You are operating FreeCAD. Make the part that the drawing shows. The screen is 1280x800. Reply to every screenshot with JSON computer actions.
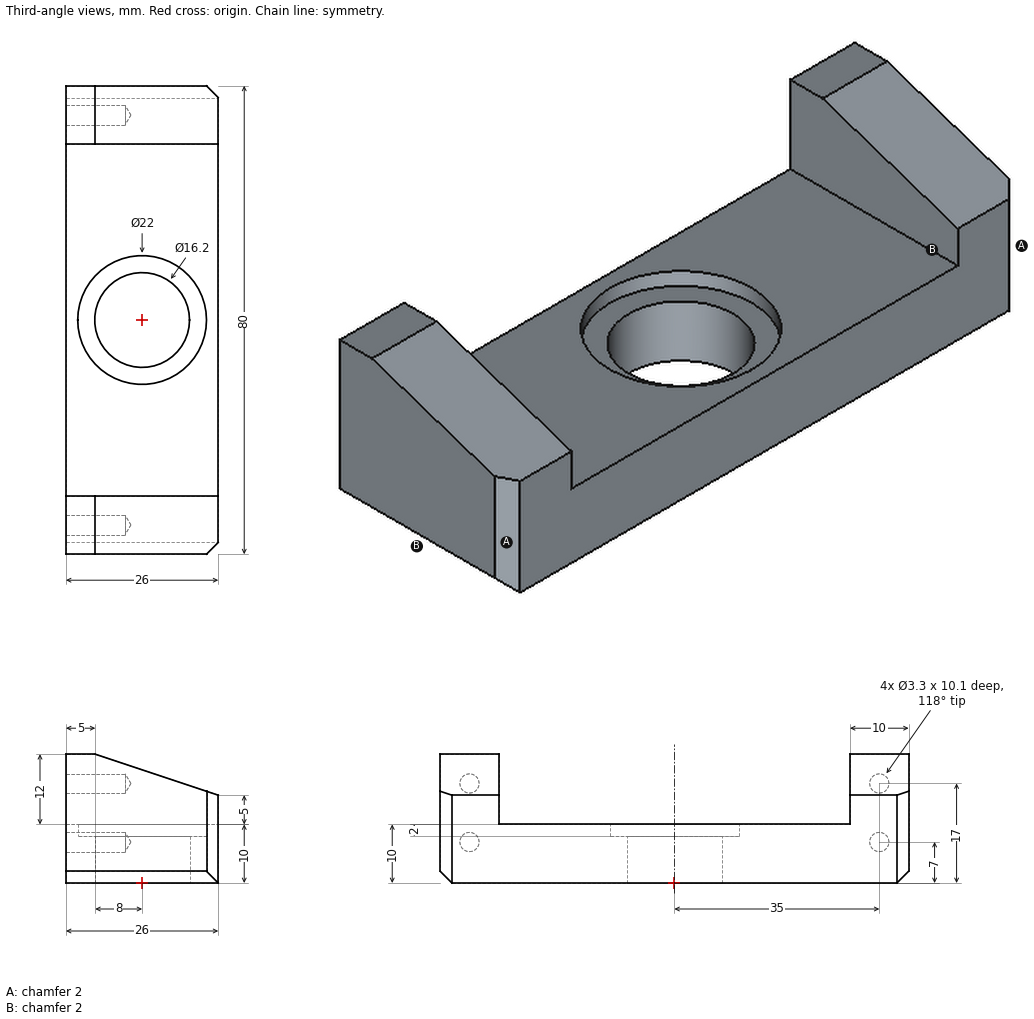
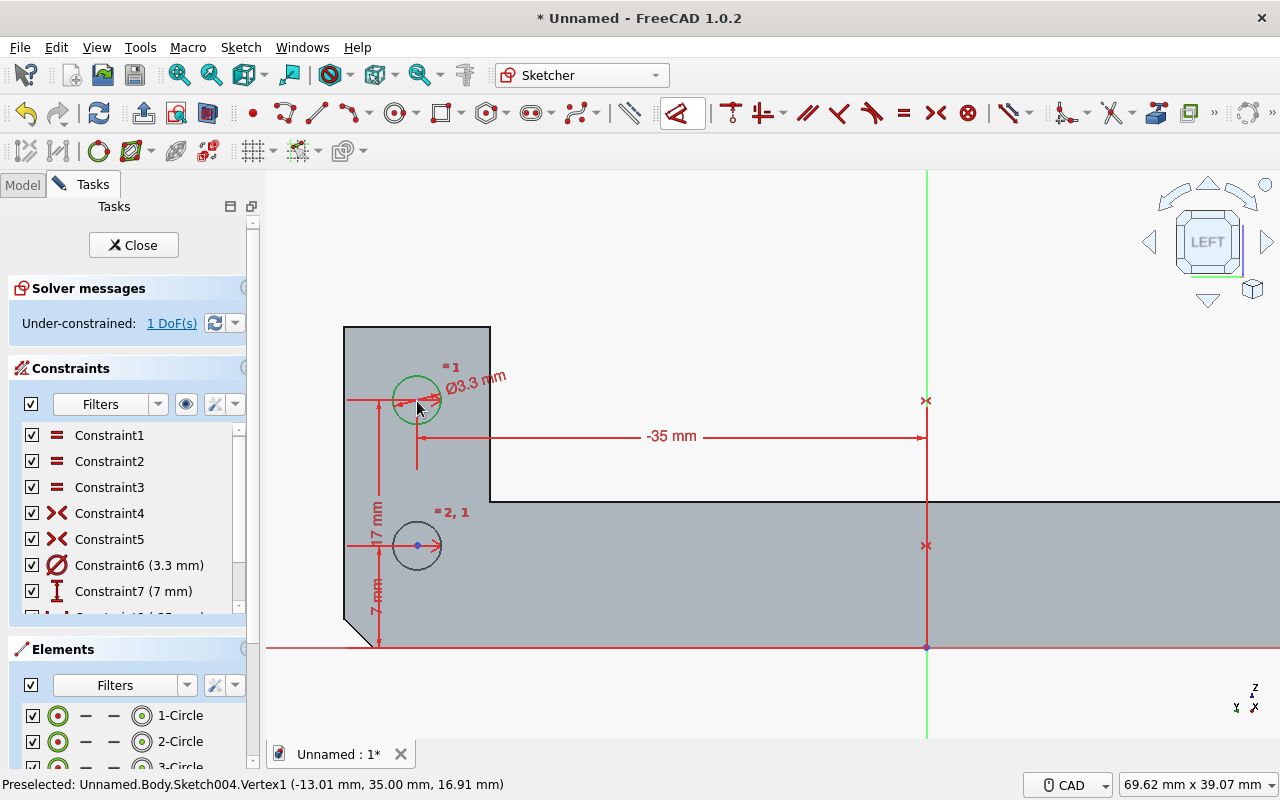
{"action": "left_click", "coordinate": [417, 546]}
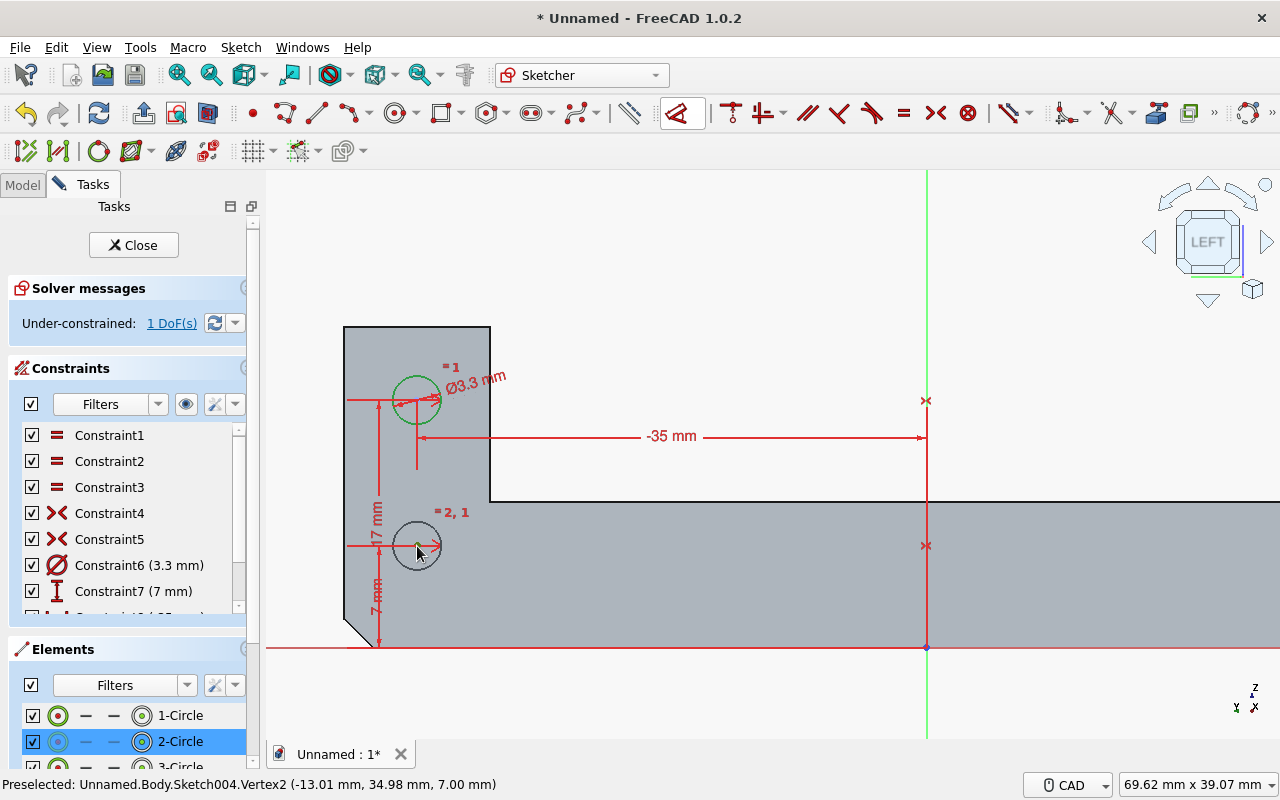
{"action": "key", "text": "l"}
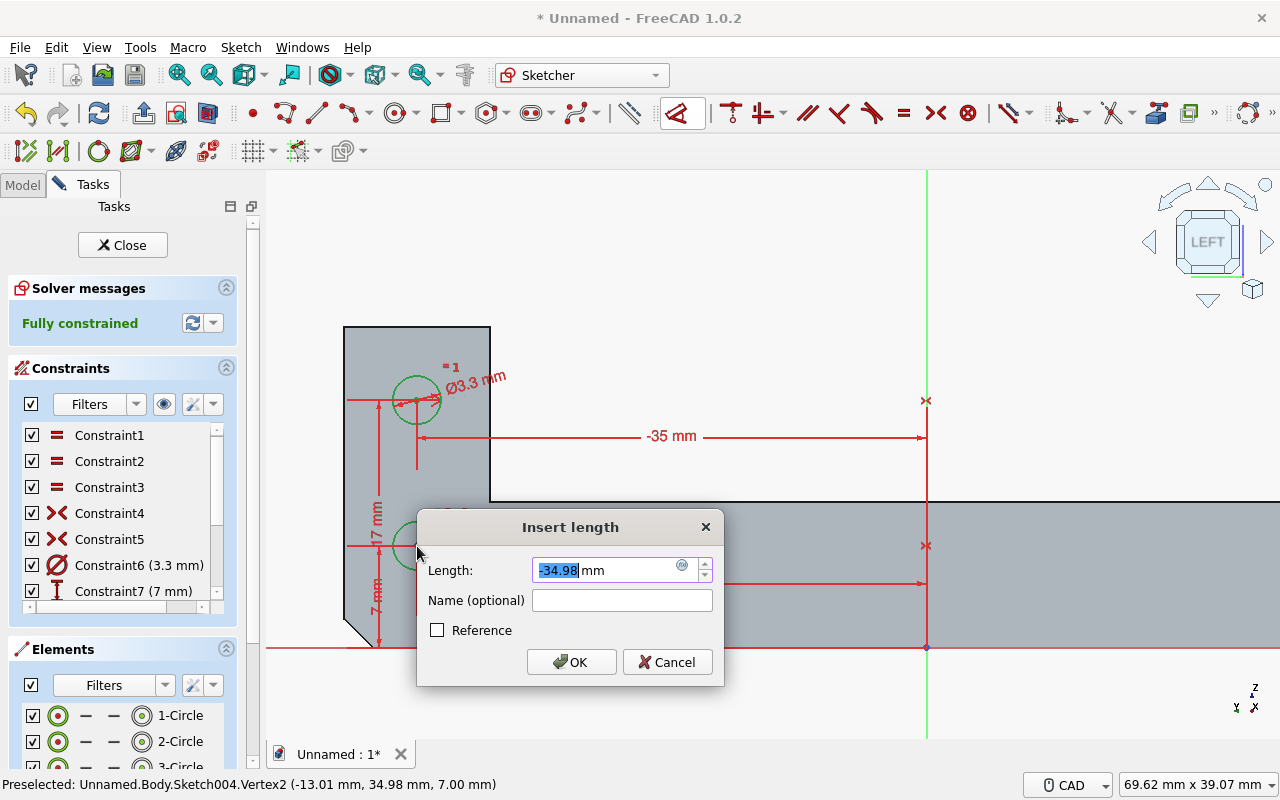
{"action": "type", "text": "-35"}
{"action": "key", "text": "Return"}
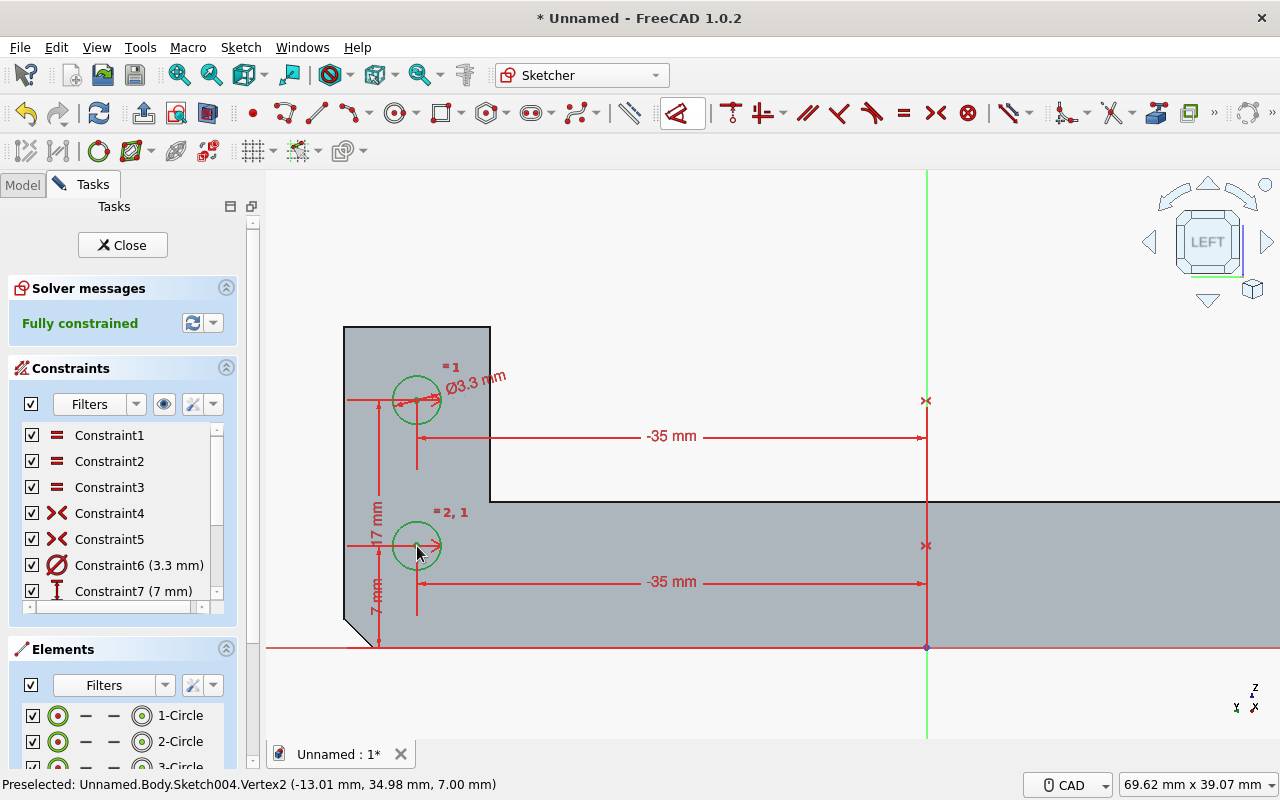
{"action": "left_click", "coordinate": [123, 245]}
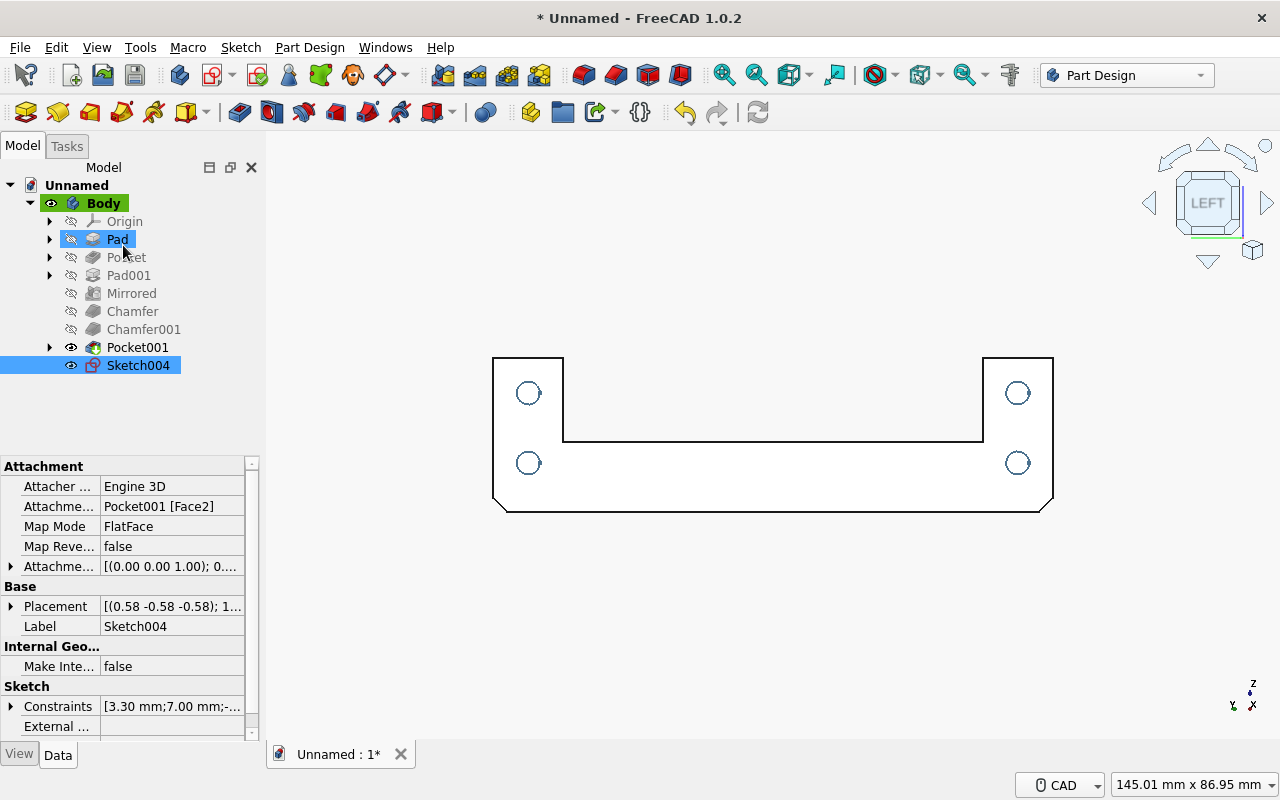
{"action": "left_click", "coordinate": [272, 112]}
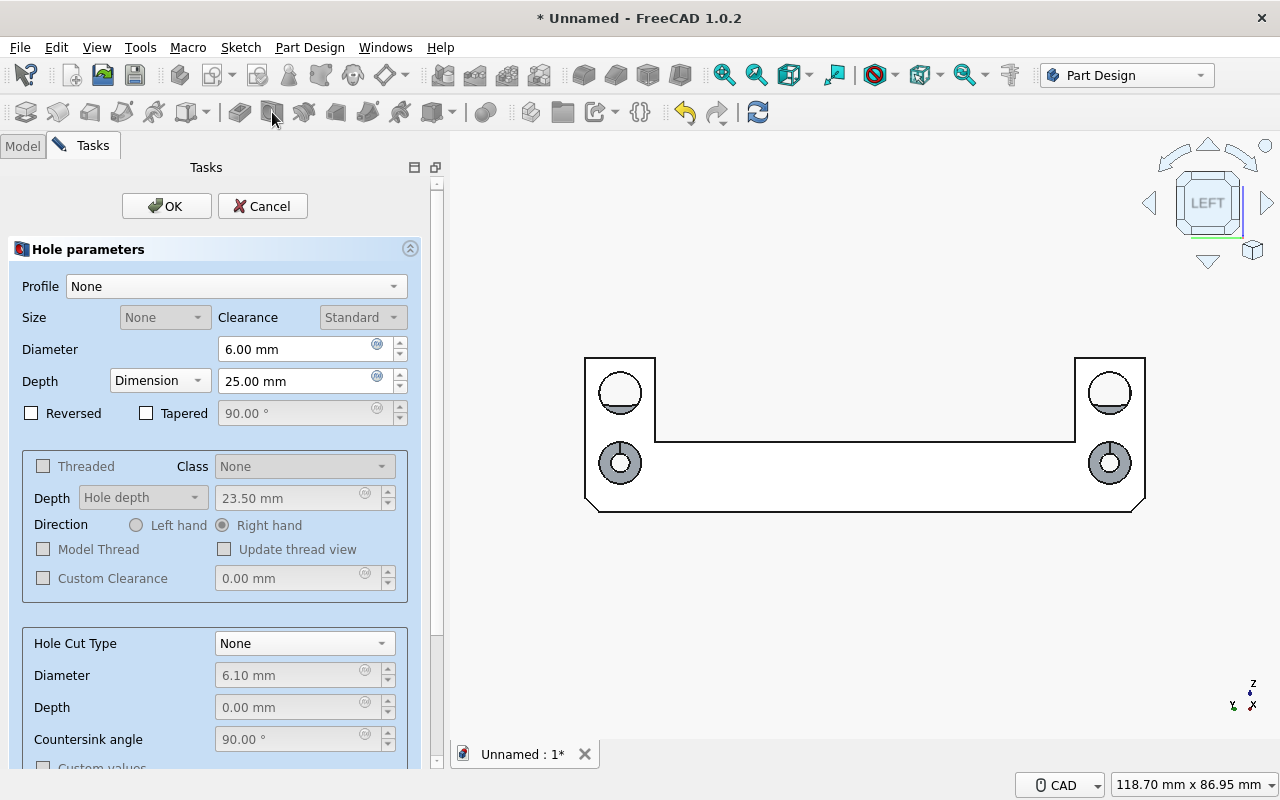
{"action": "triple_click", "coordinate": [305, 349]}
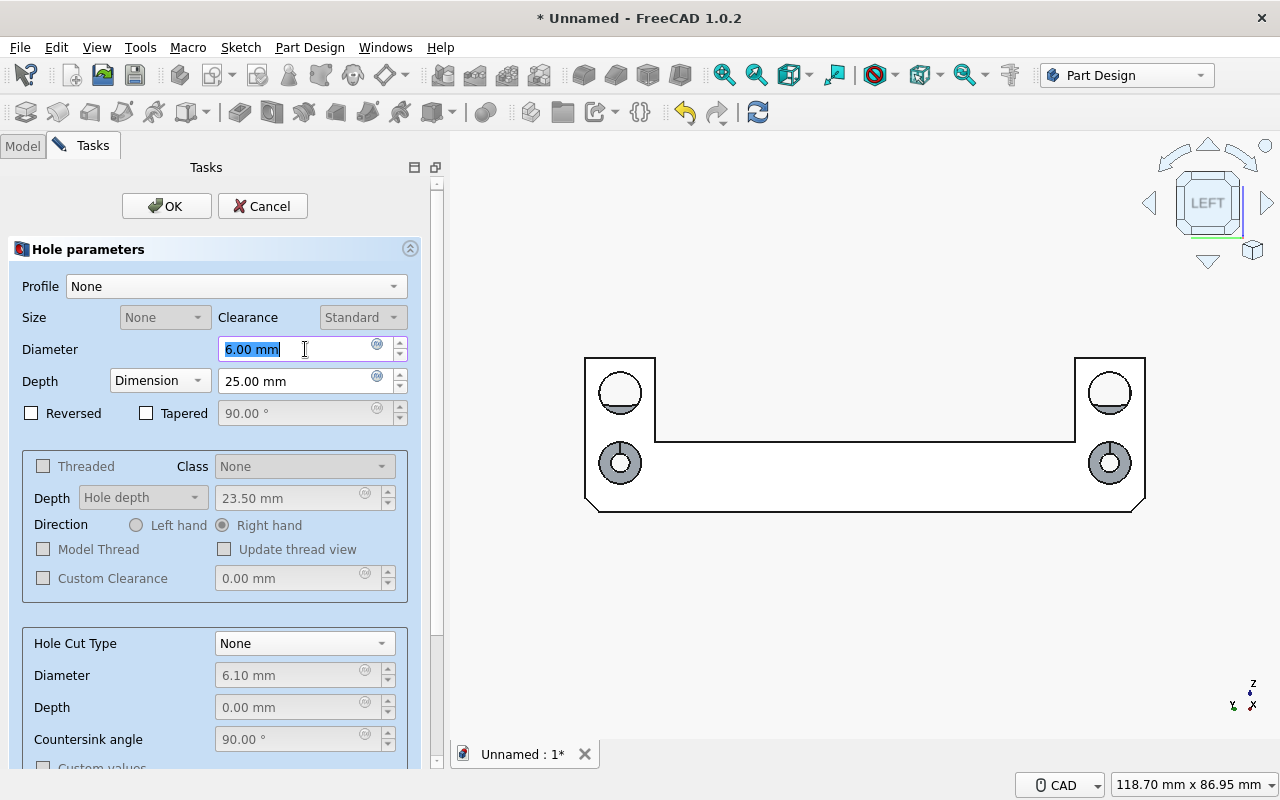
{"action": "type", "text": "3.3"}
{"action": "key", "text": "Tab"}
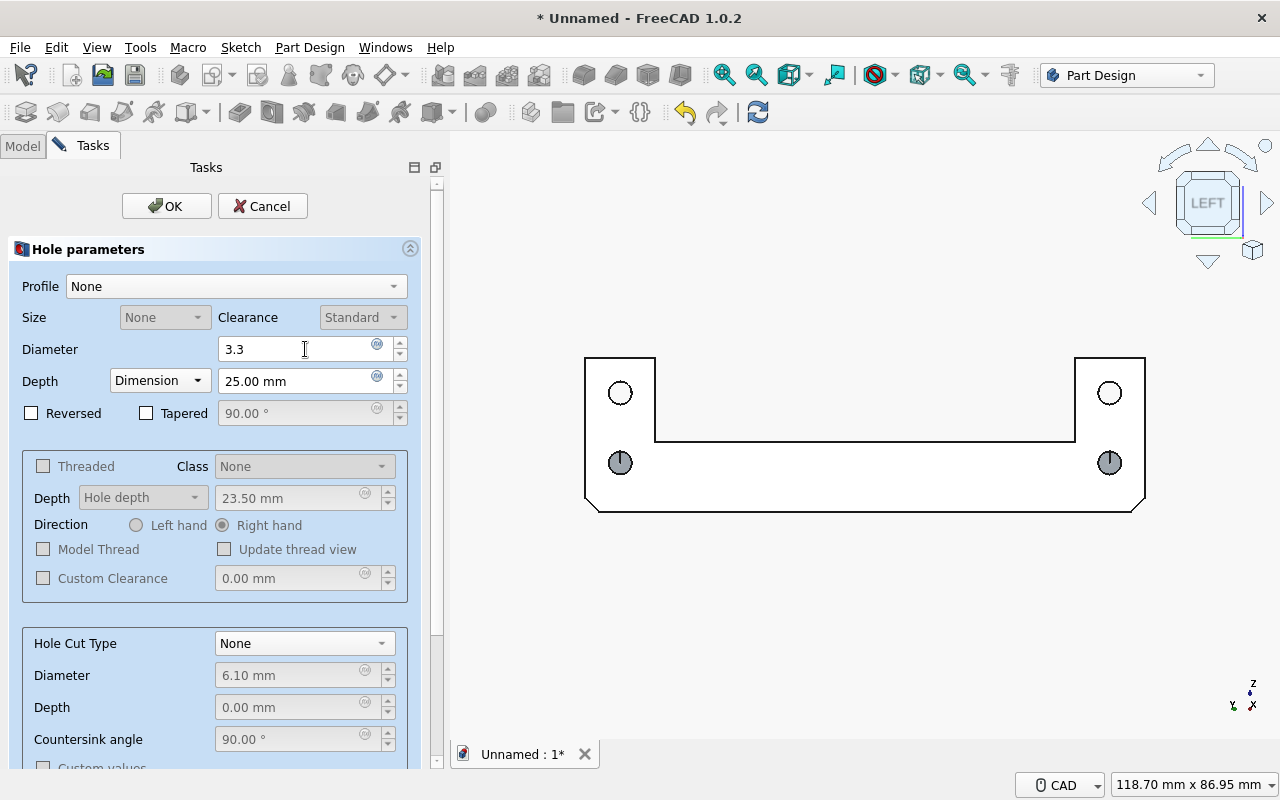
{"action": "triple_click", "coordinate": [305, 381]}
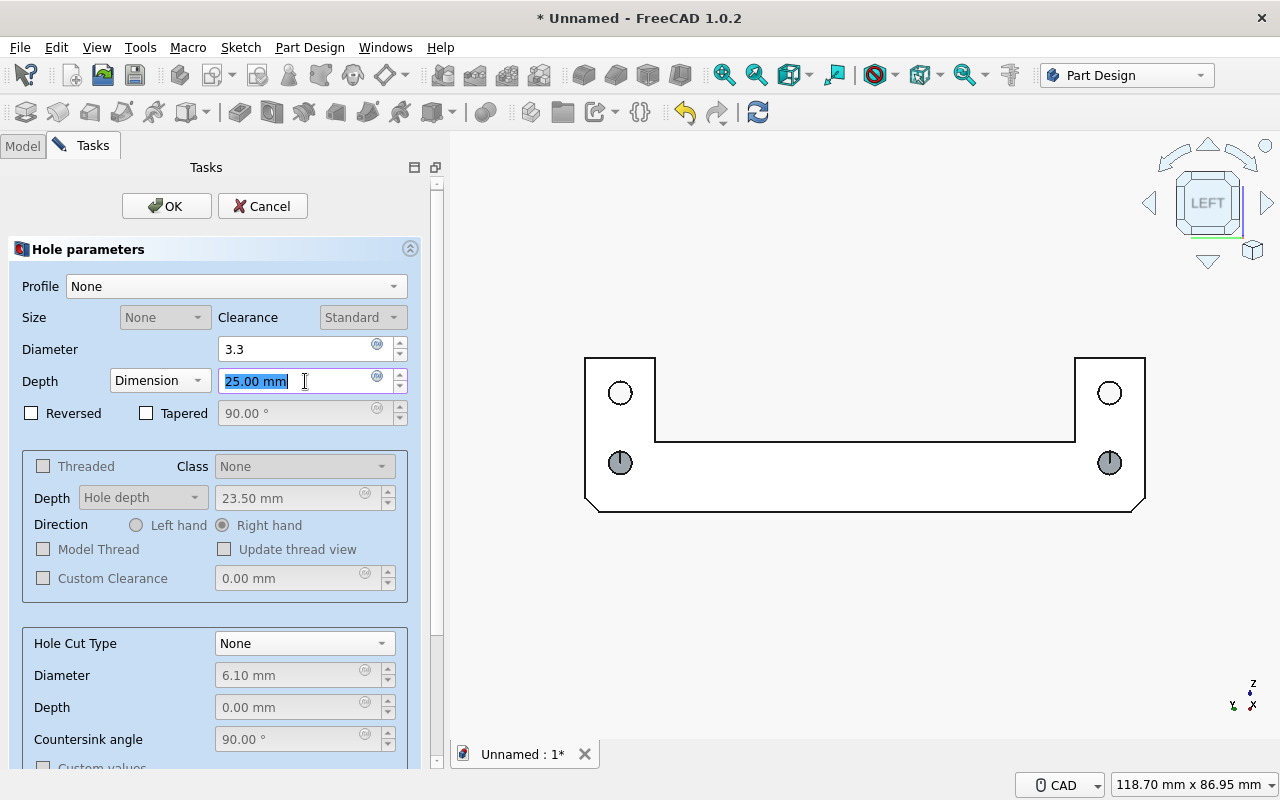
{"action": "type", "text": "10.1"}
{"action": "key", "text": "Tab"}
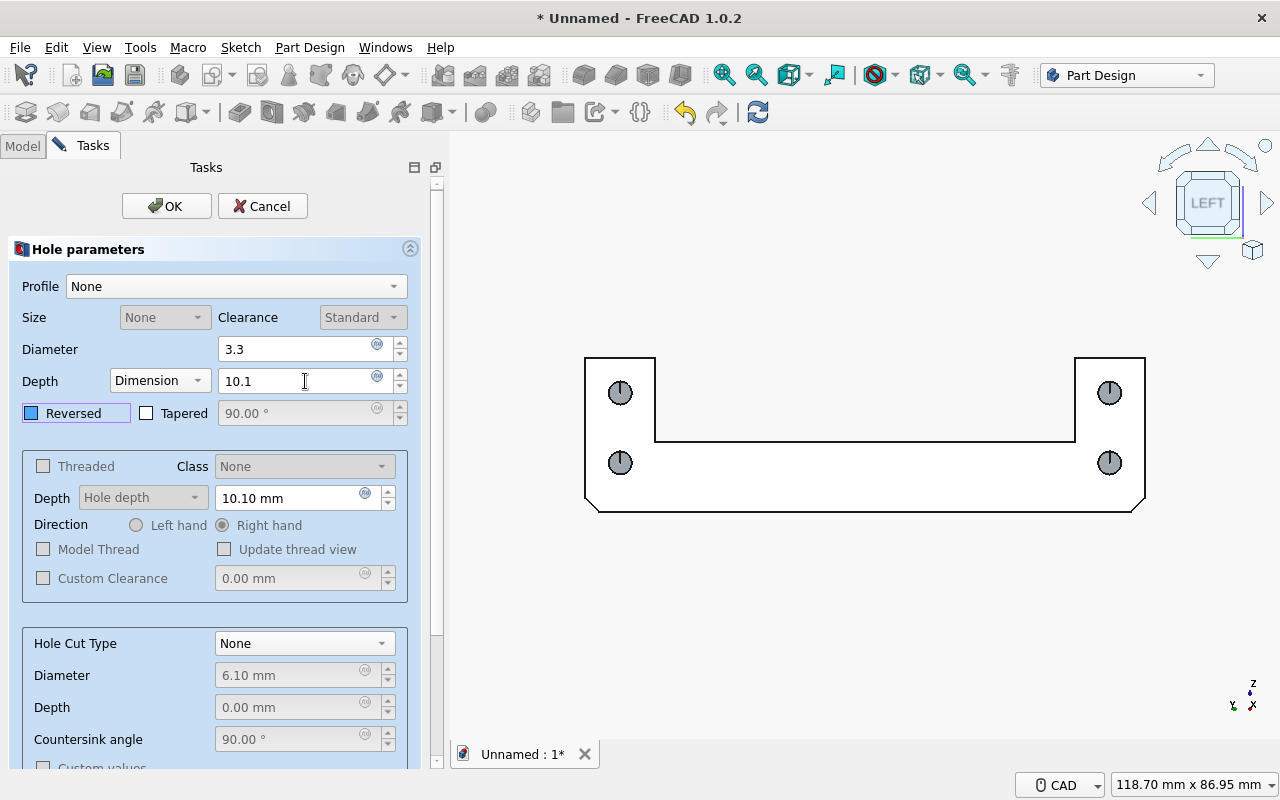
{"action": "left_click", "coordinate": [167, 206]}